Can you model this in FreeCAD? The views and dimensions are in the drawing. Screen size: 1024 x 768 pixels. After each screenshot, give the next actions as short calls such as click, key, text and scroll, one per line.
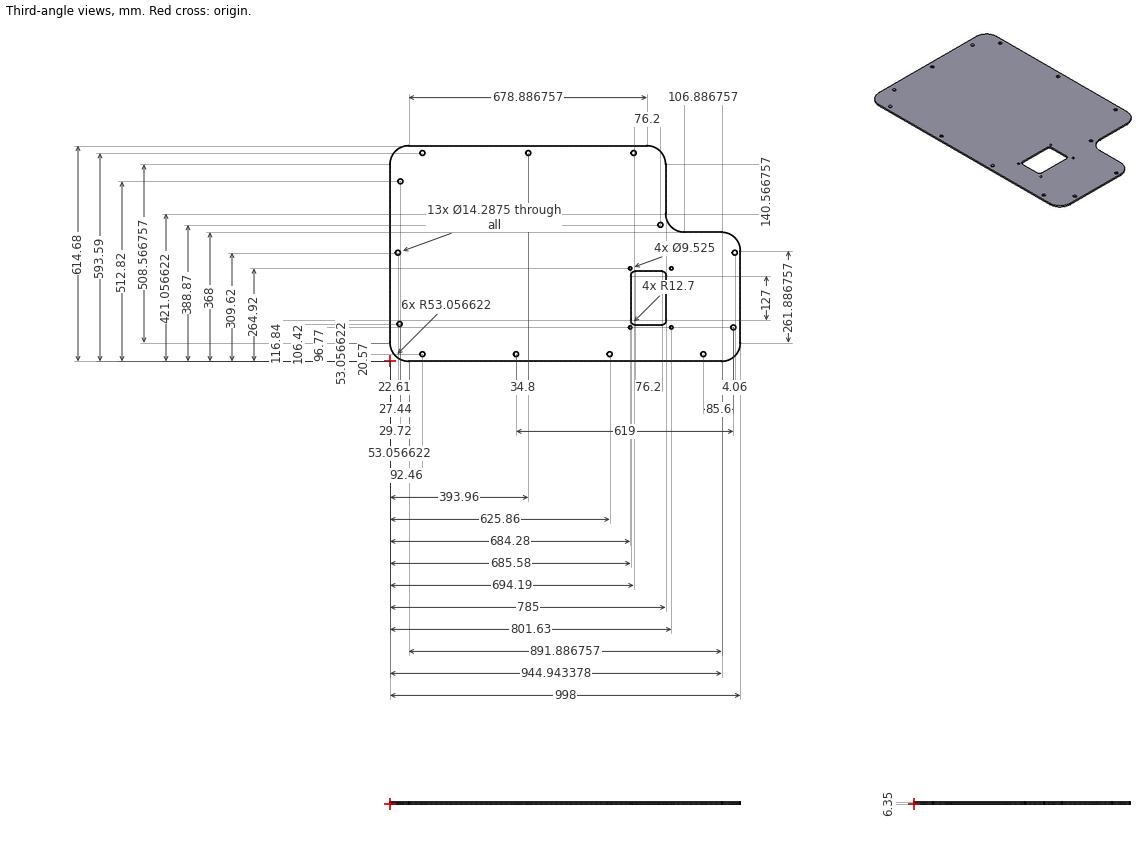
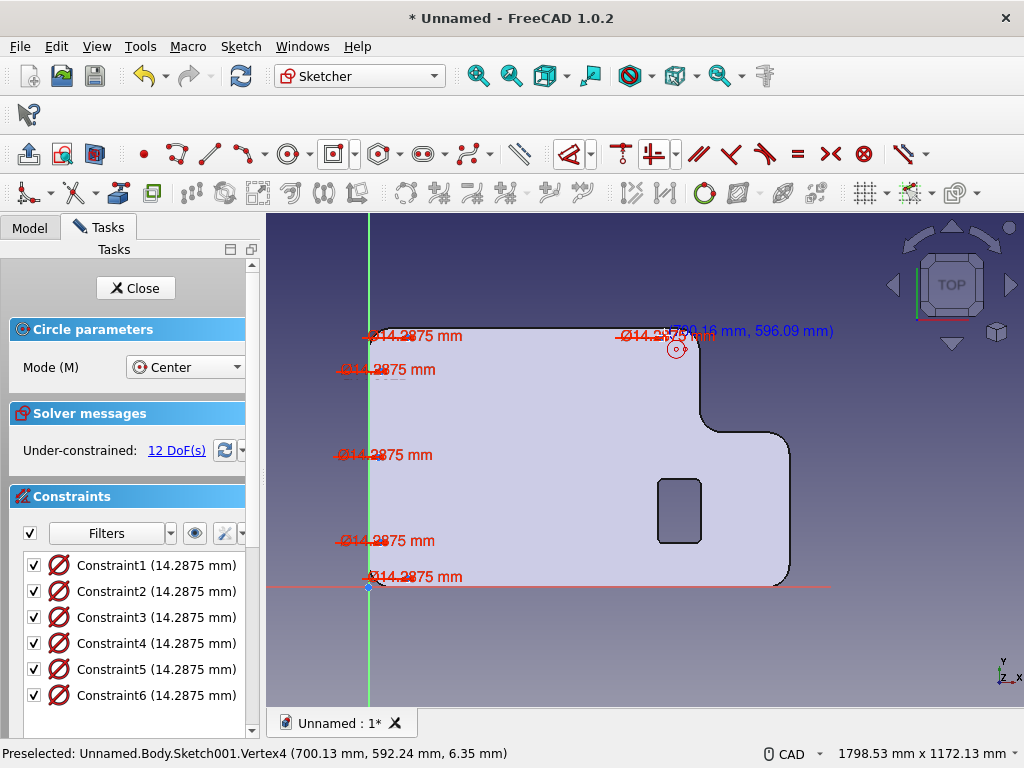
scroll(535, 337, up, 11)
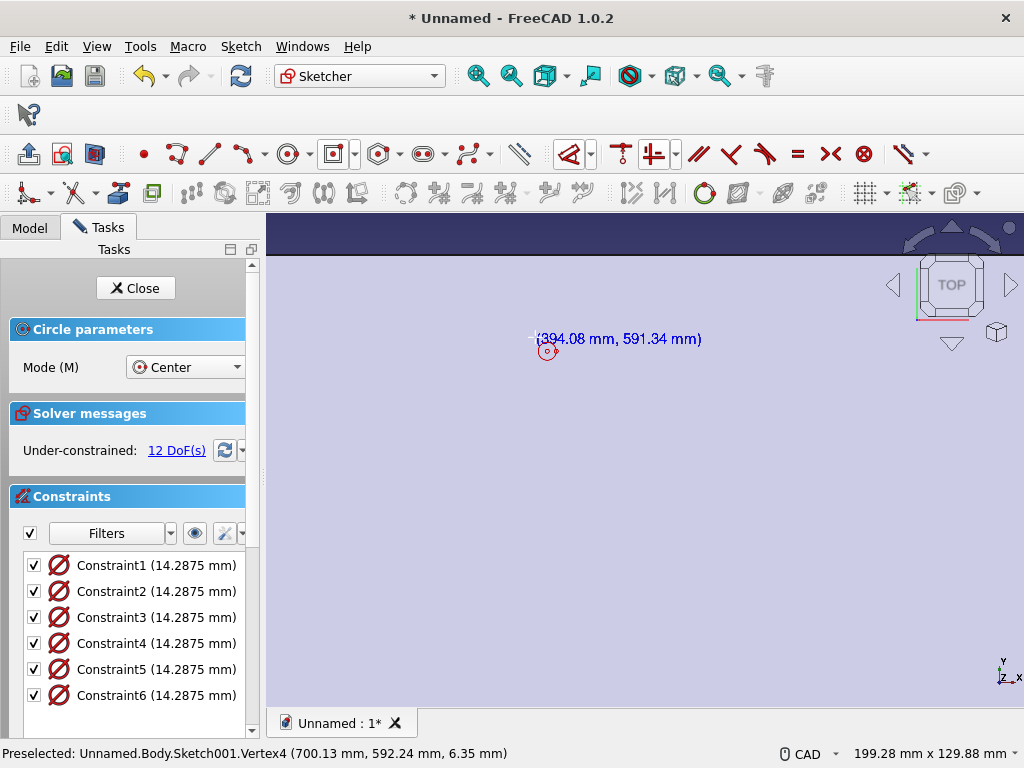
scroll(534, 337, down, 11)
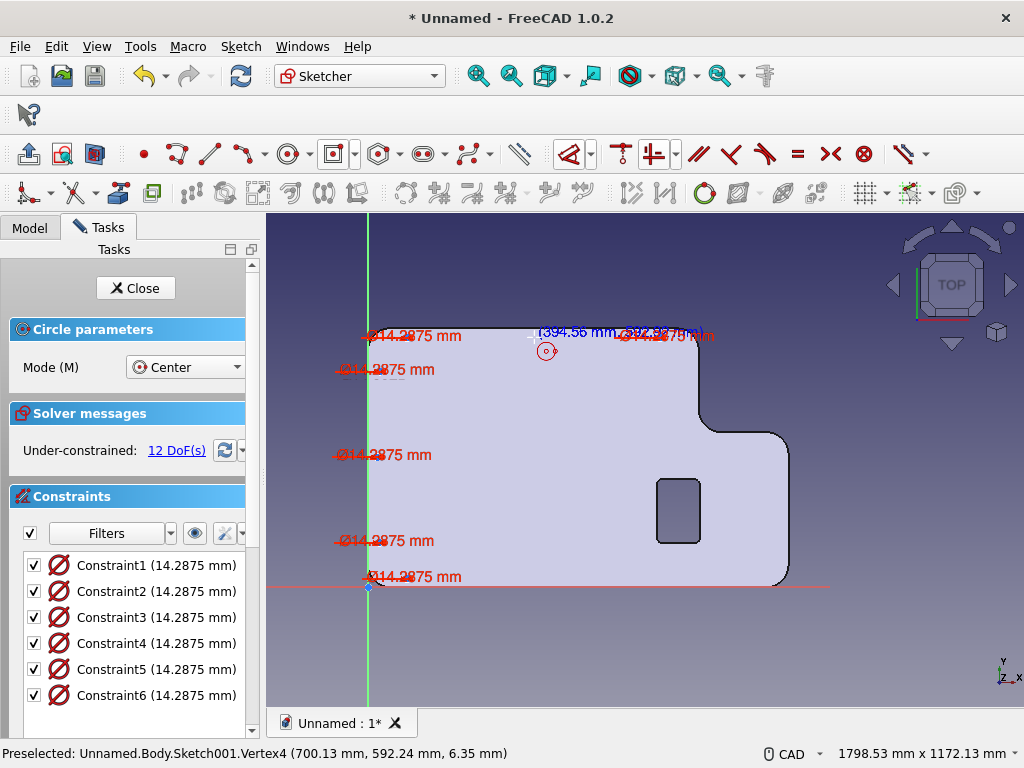
click(534, 337)
move(536, 335)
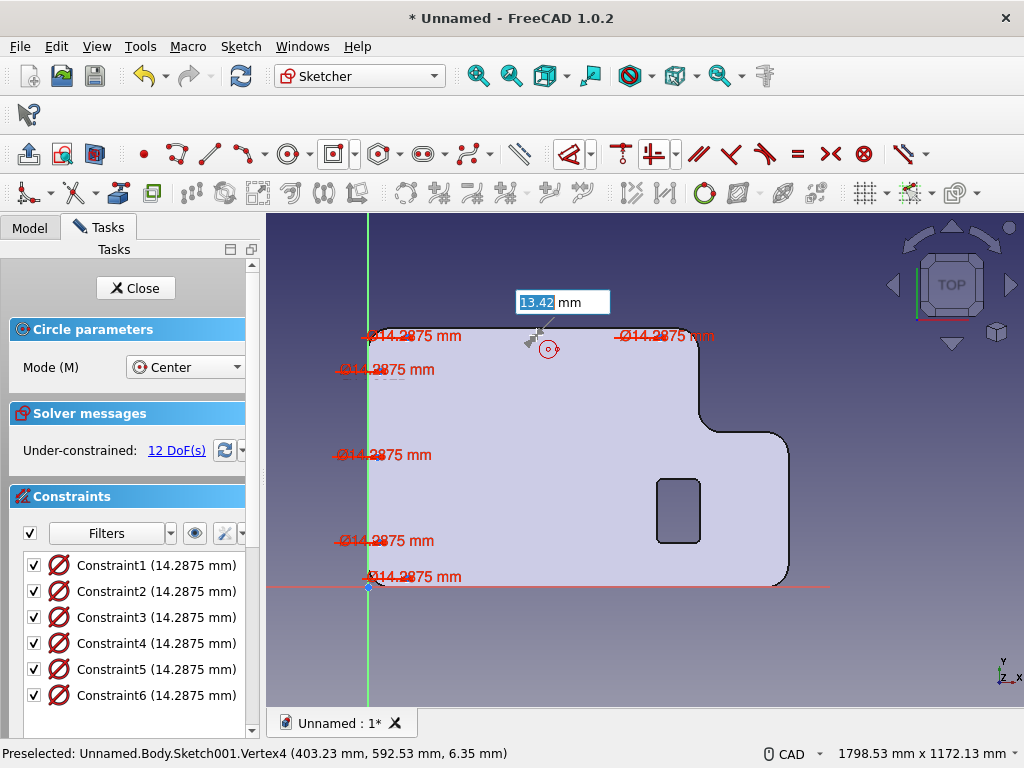
text(14.2875)
key(Return)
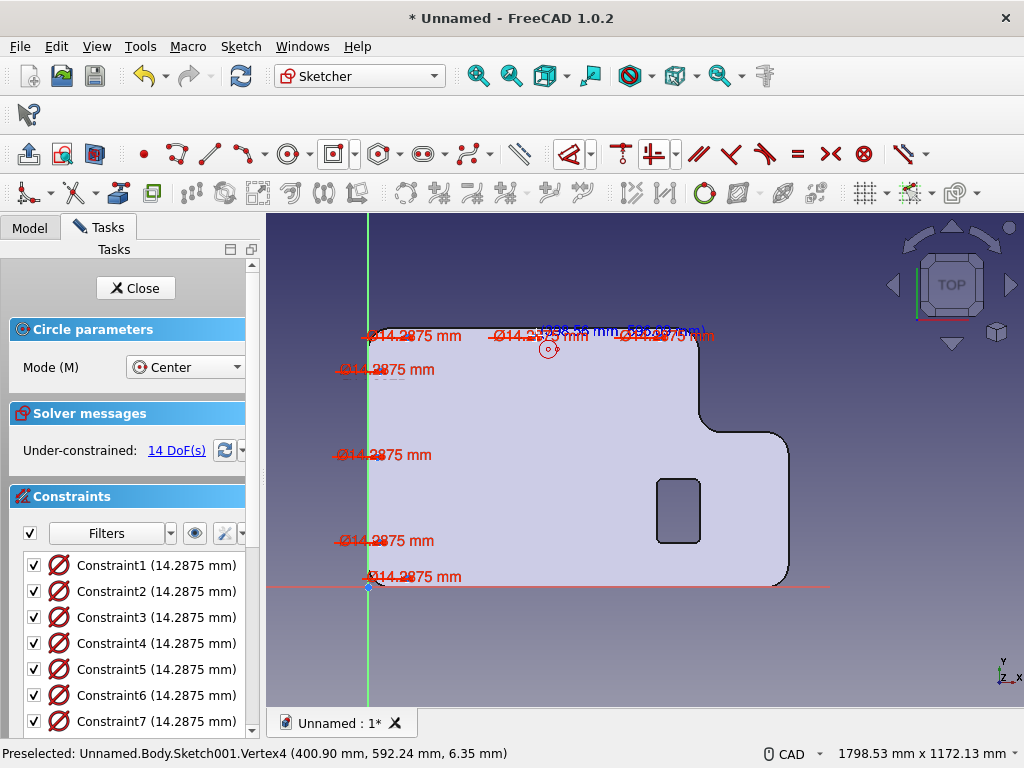
scroll(519, 579, up, 11)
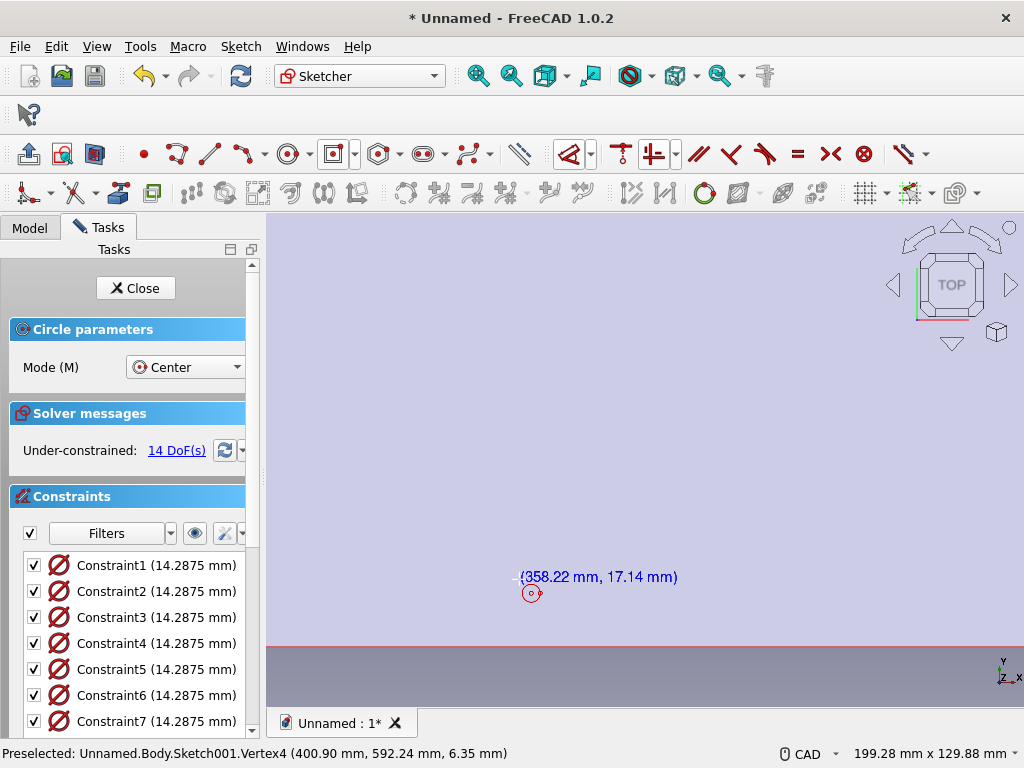
scroll(519, 579, down, 11)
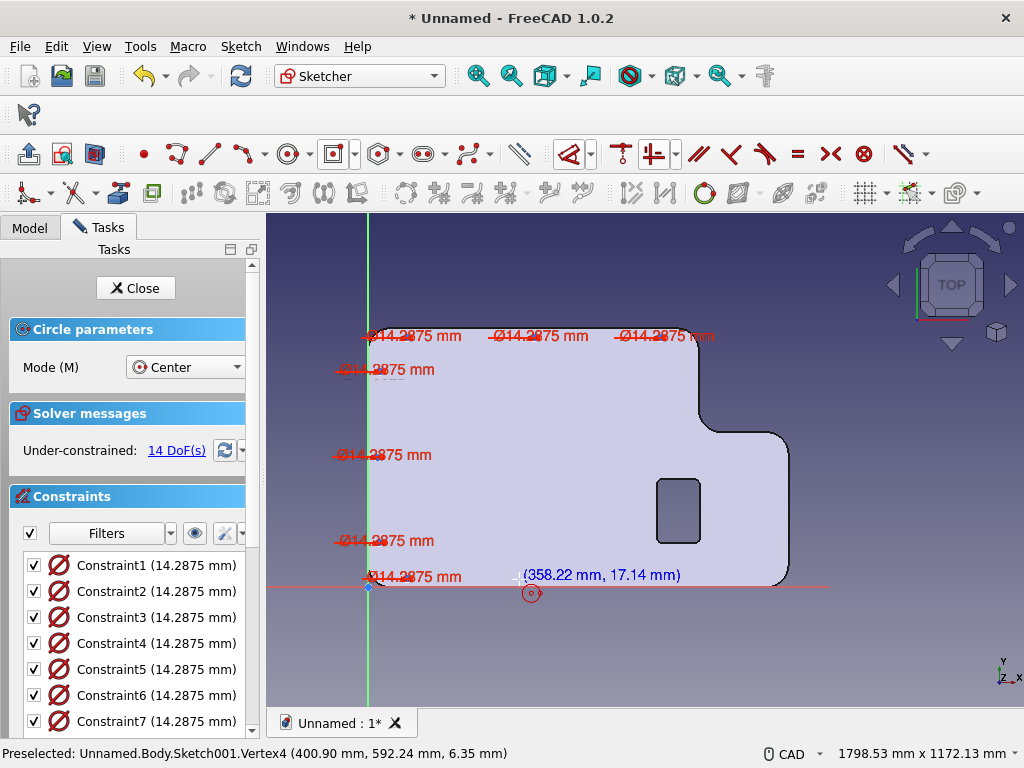
scroll(519, 579, up, 4)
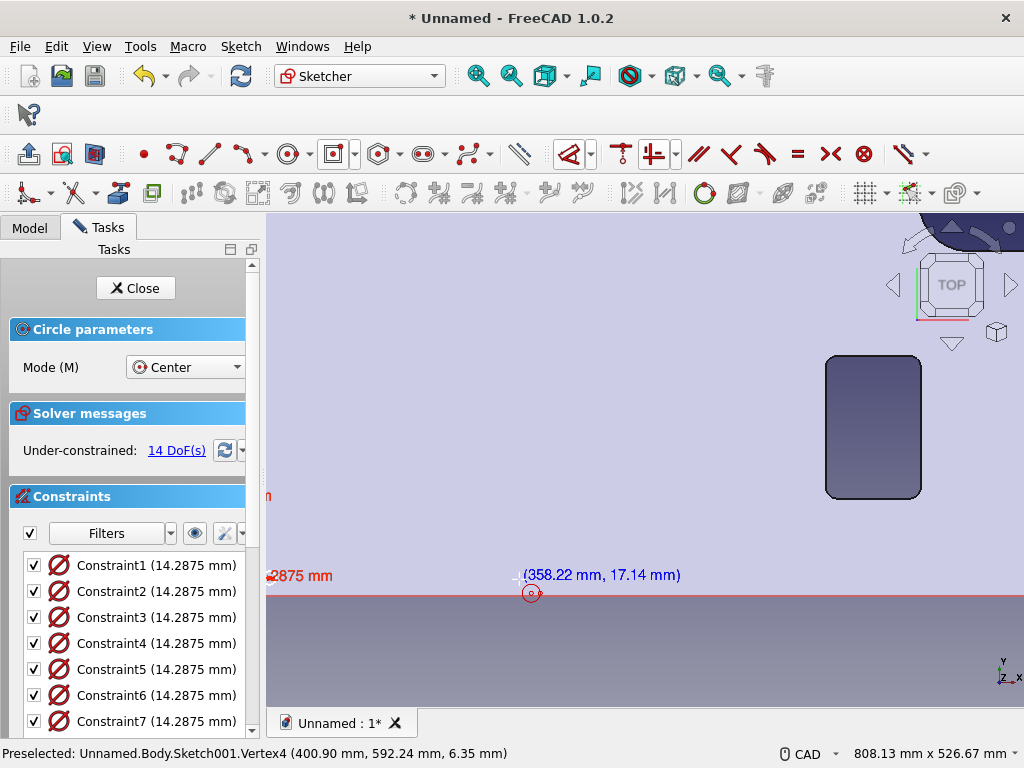
click(519, 577)
move(524, 572)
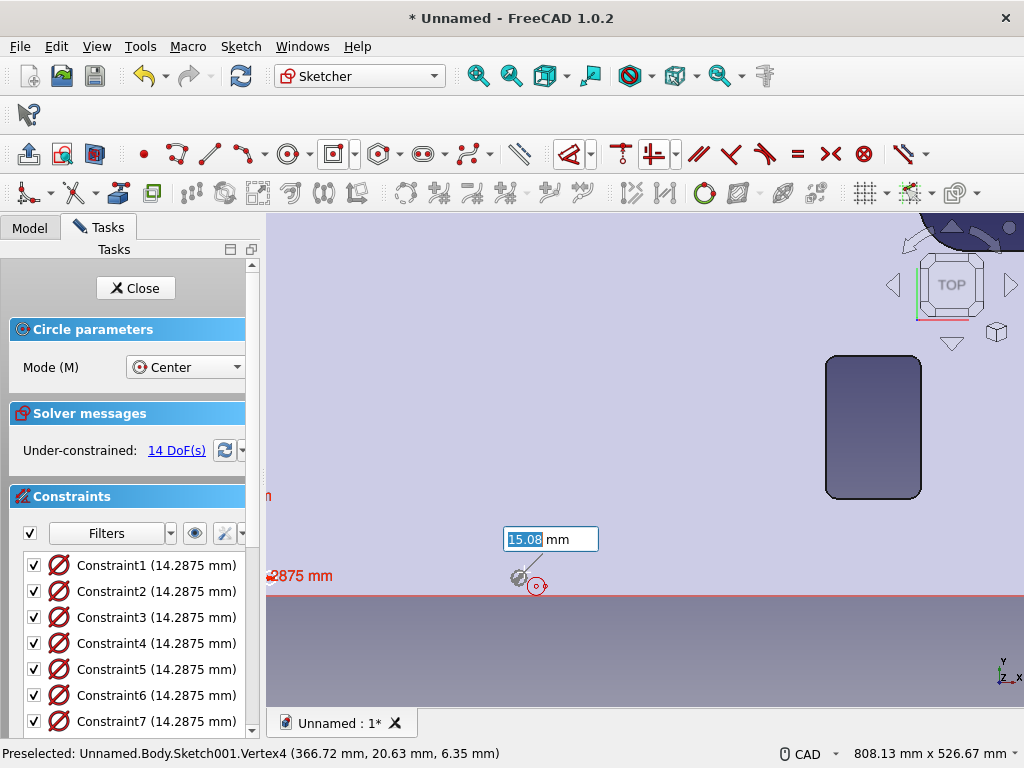
text(14.2875)
key(Return)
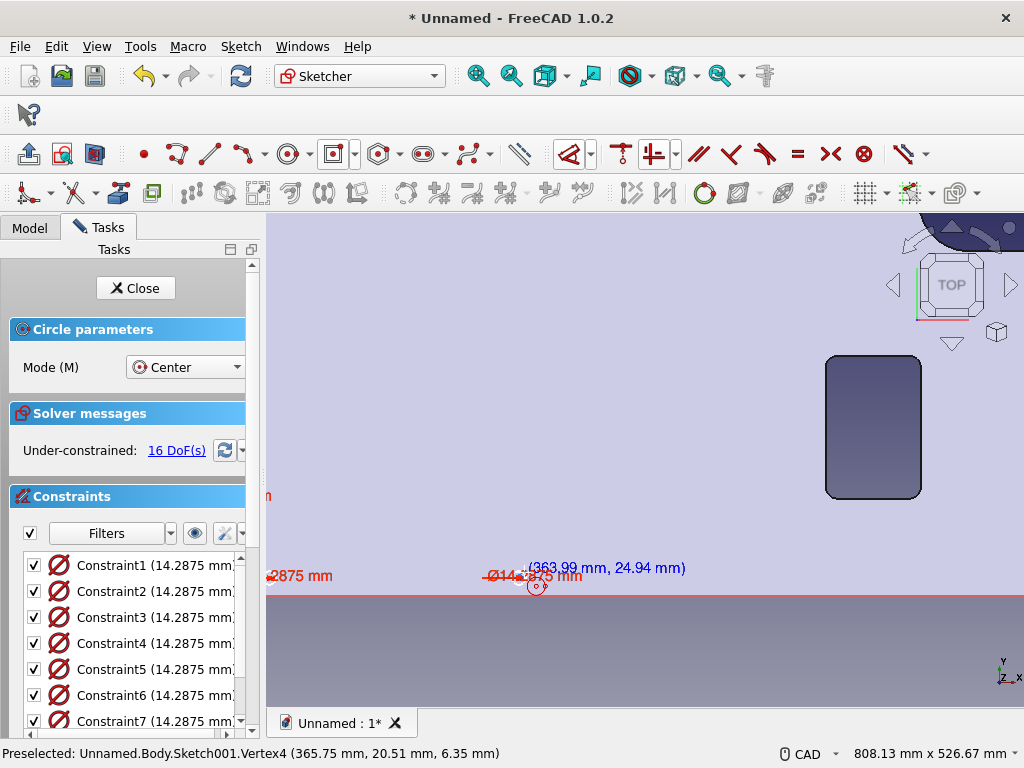
scroll(770, 577, up, 7)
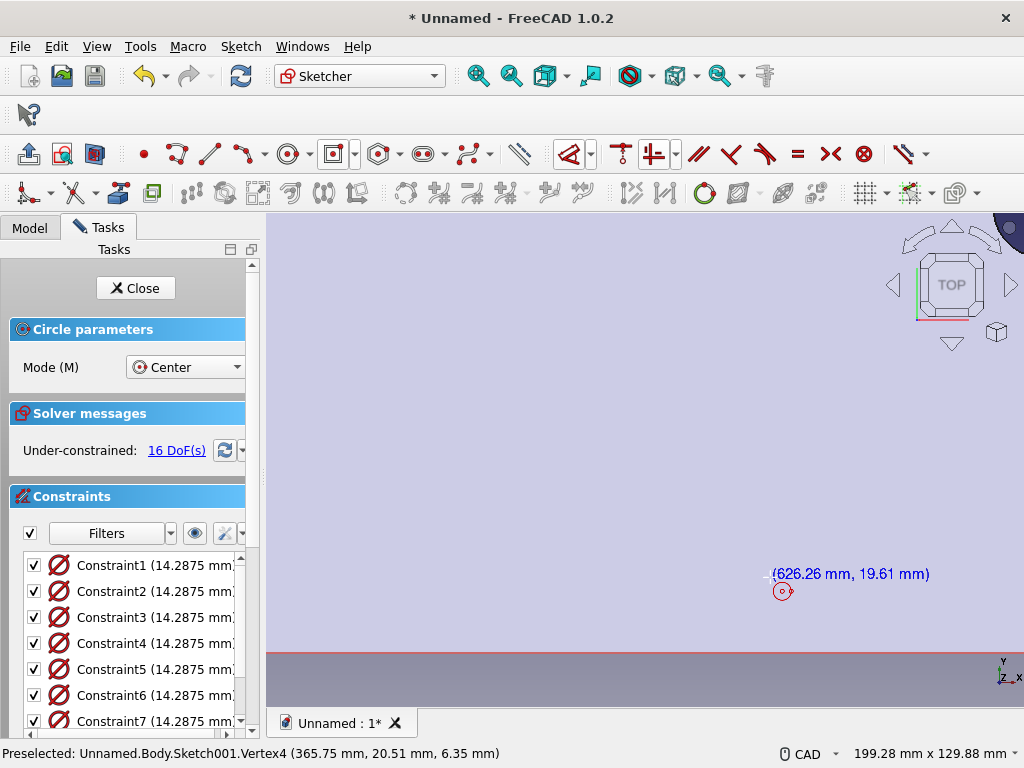
scroll(615, 578, down, 11)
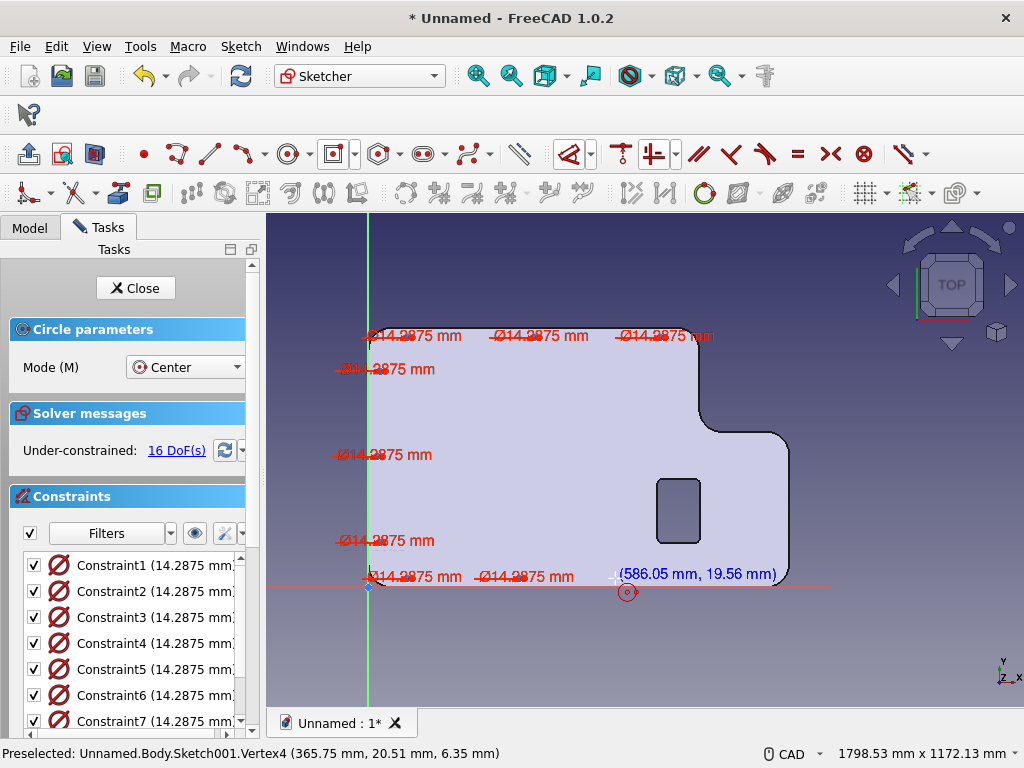
scroll(632, 578, up, 4)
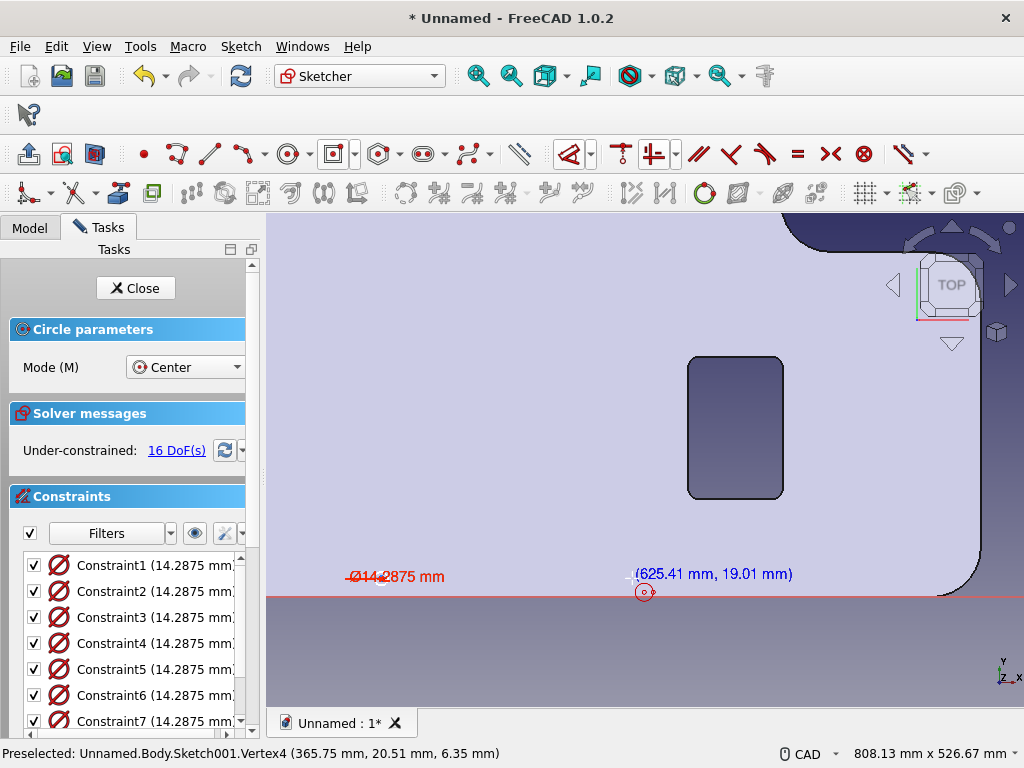
click(632, 578)
move(637, 573)